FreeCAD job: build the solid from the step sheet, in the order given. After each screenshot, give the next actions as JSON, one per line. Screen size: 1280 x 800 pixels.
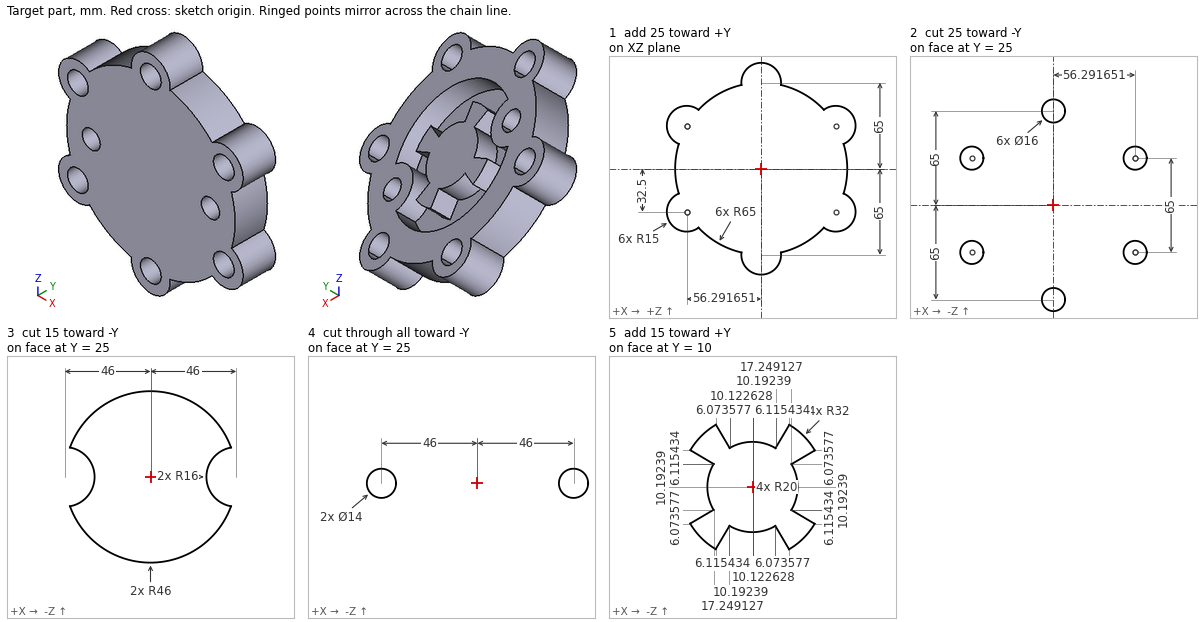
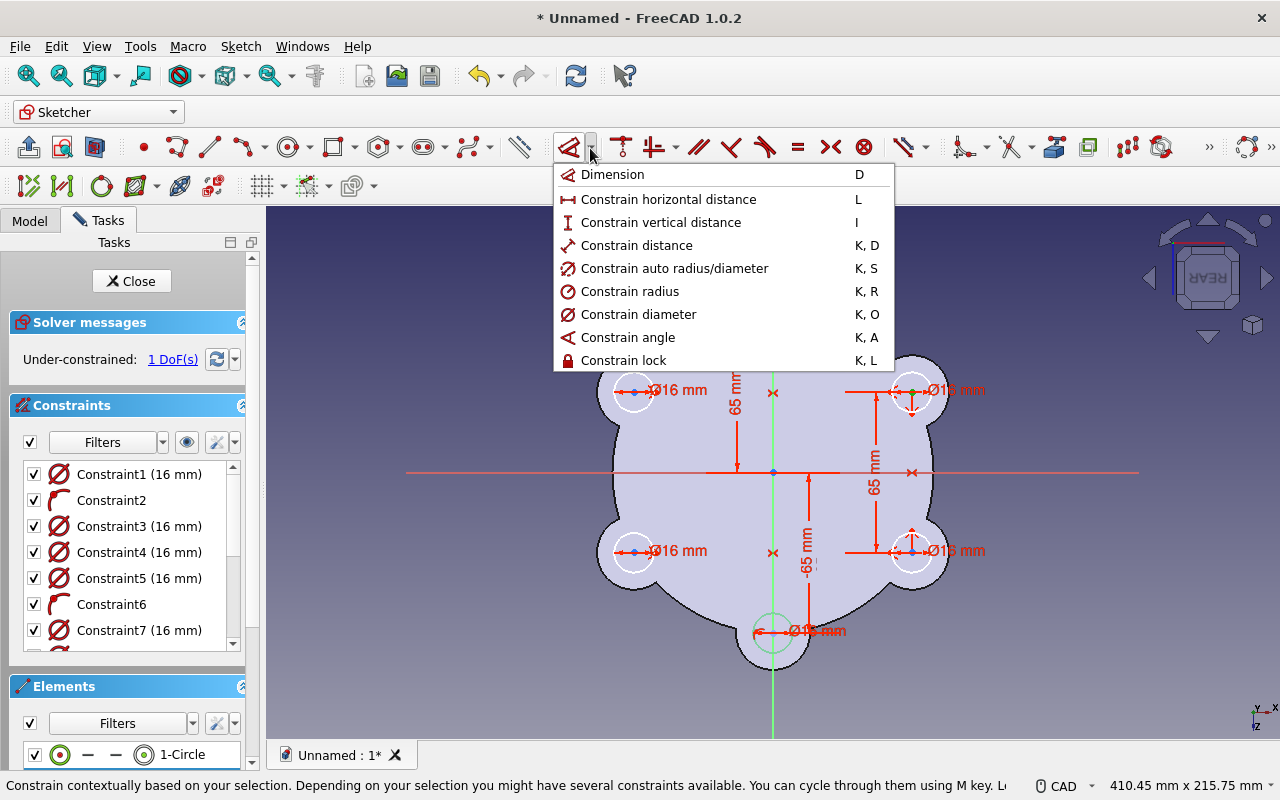
{"action": "left_click", "coordinate": [724, 200]}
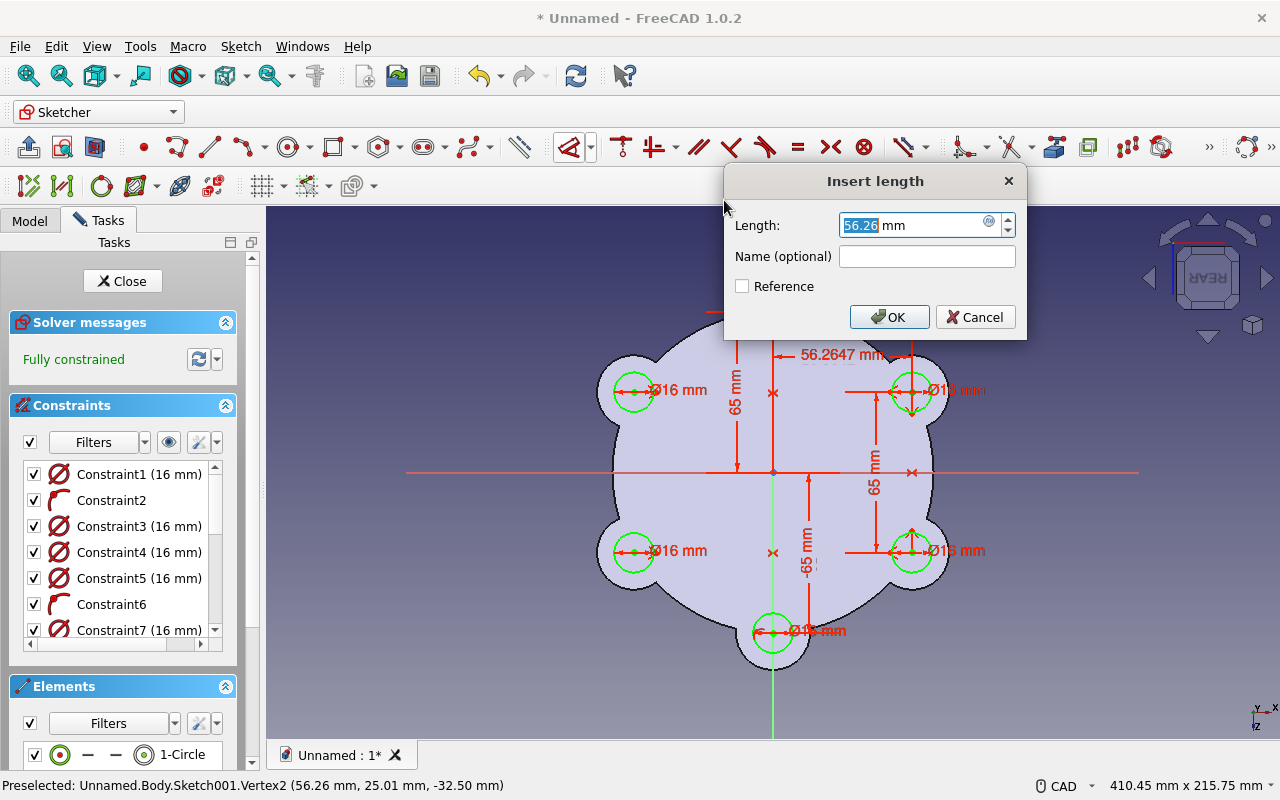
{"action": "type", "text": "56.291651"}
{"action": "key", "text": "Return"}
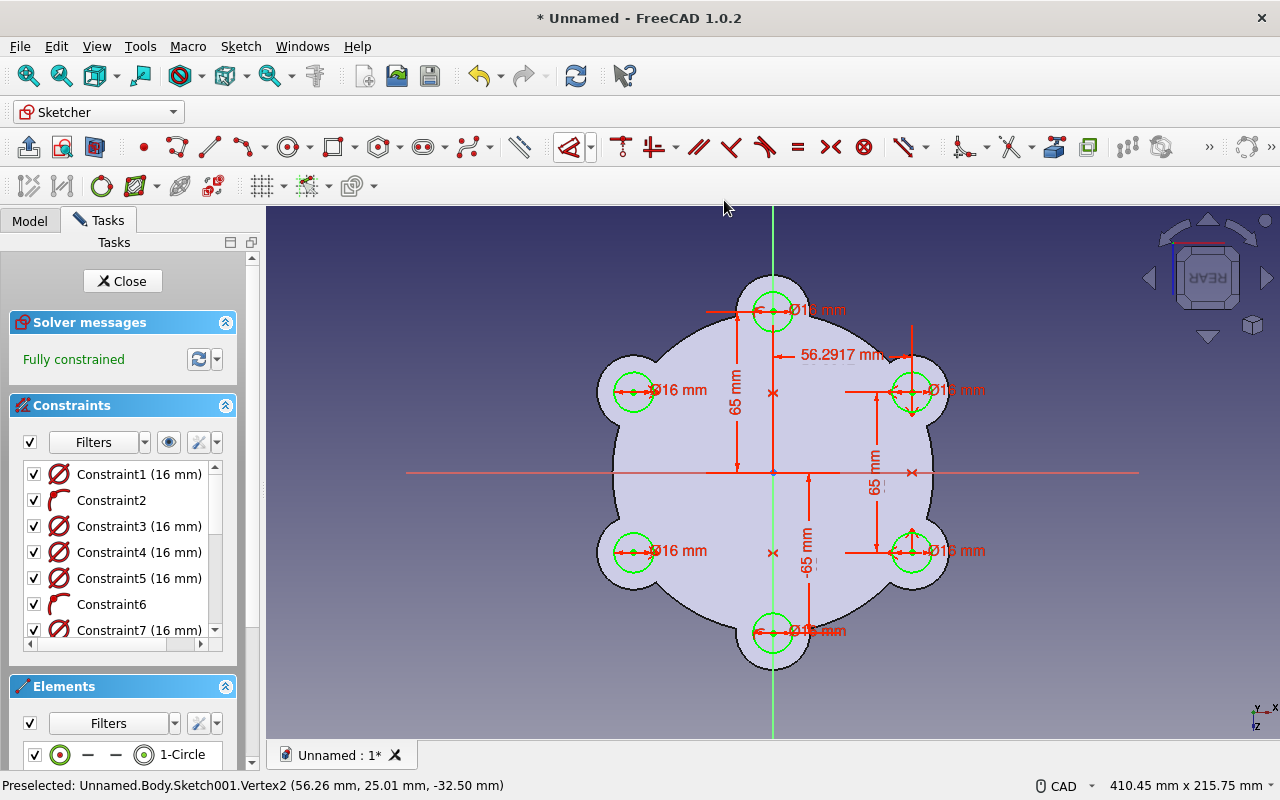
{"action": "left_click", "coordinate": [123, 281]}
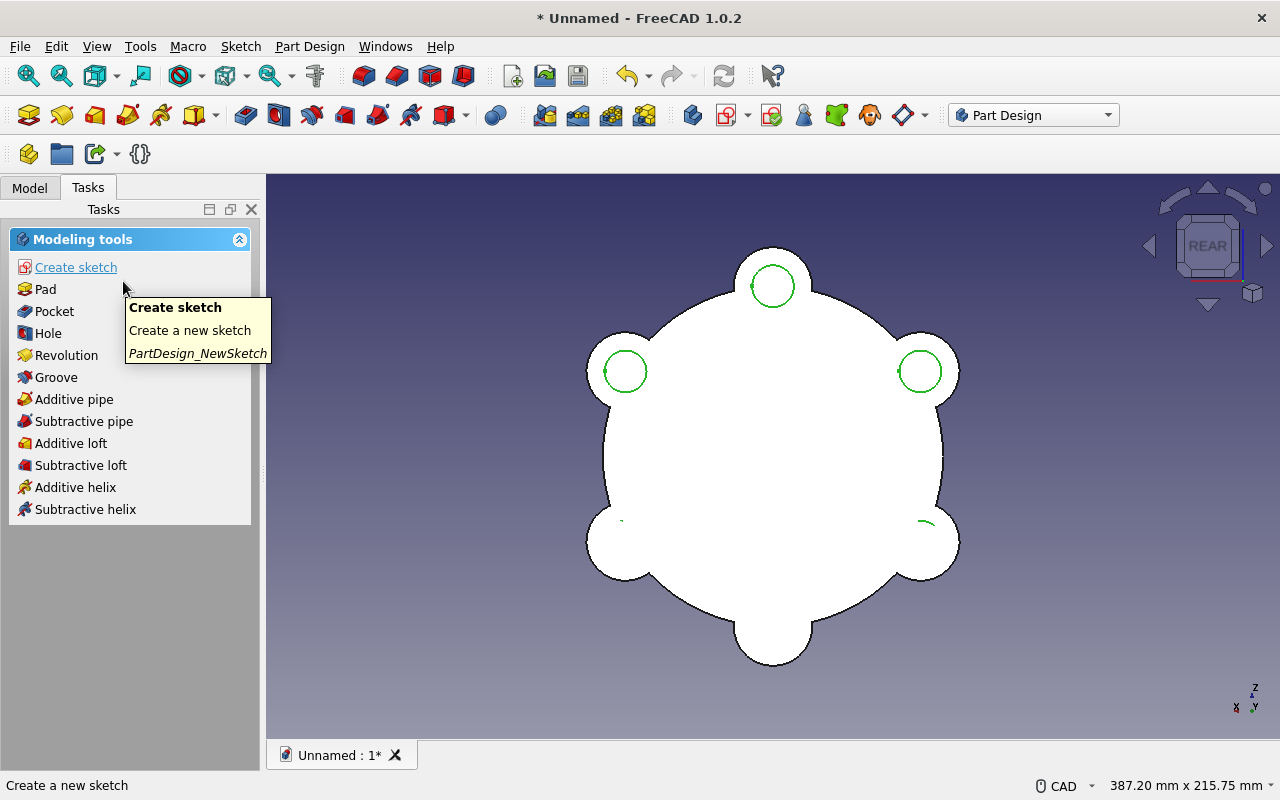
{"action": "left_click", "coordinate": [246, 116]}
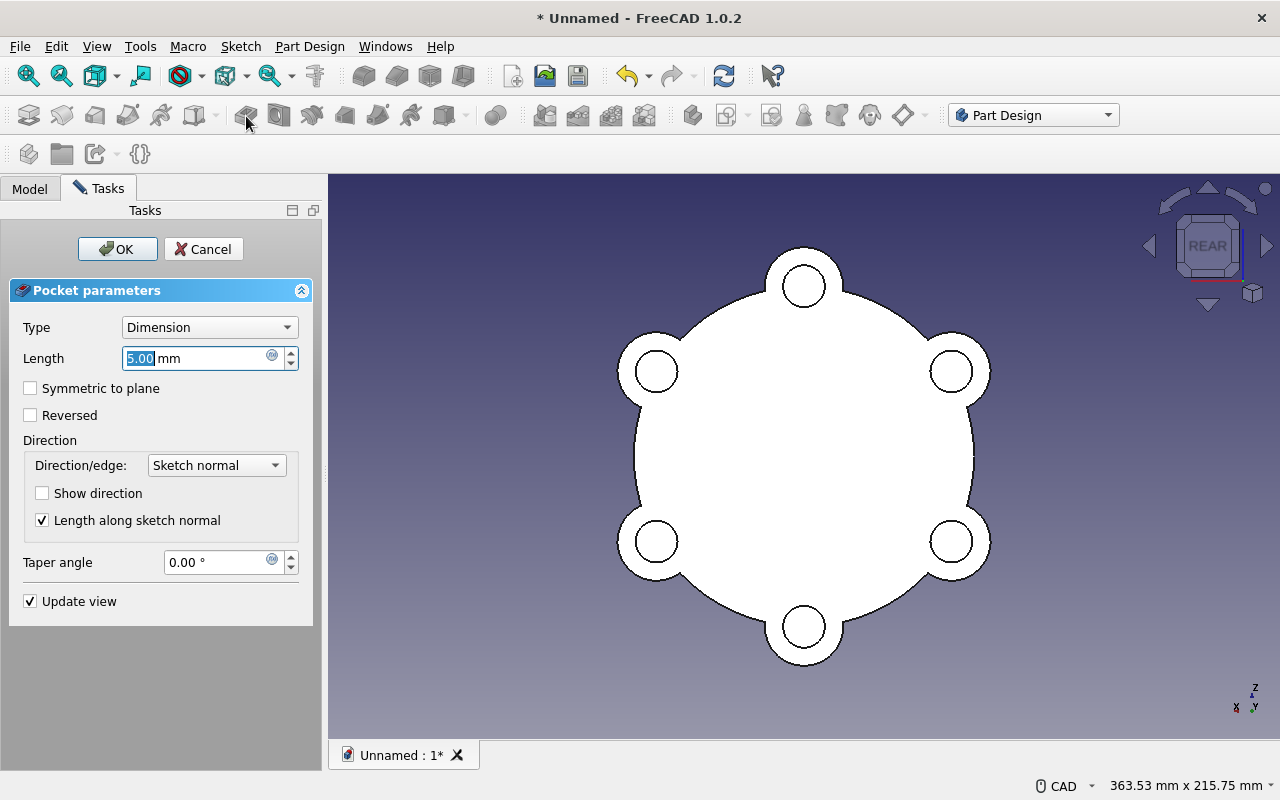
{"action": "type", "text": "25"}
{"action": "key", "text": "Tab"}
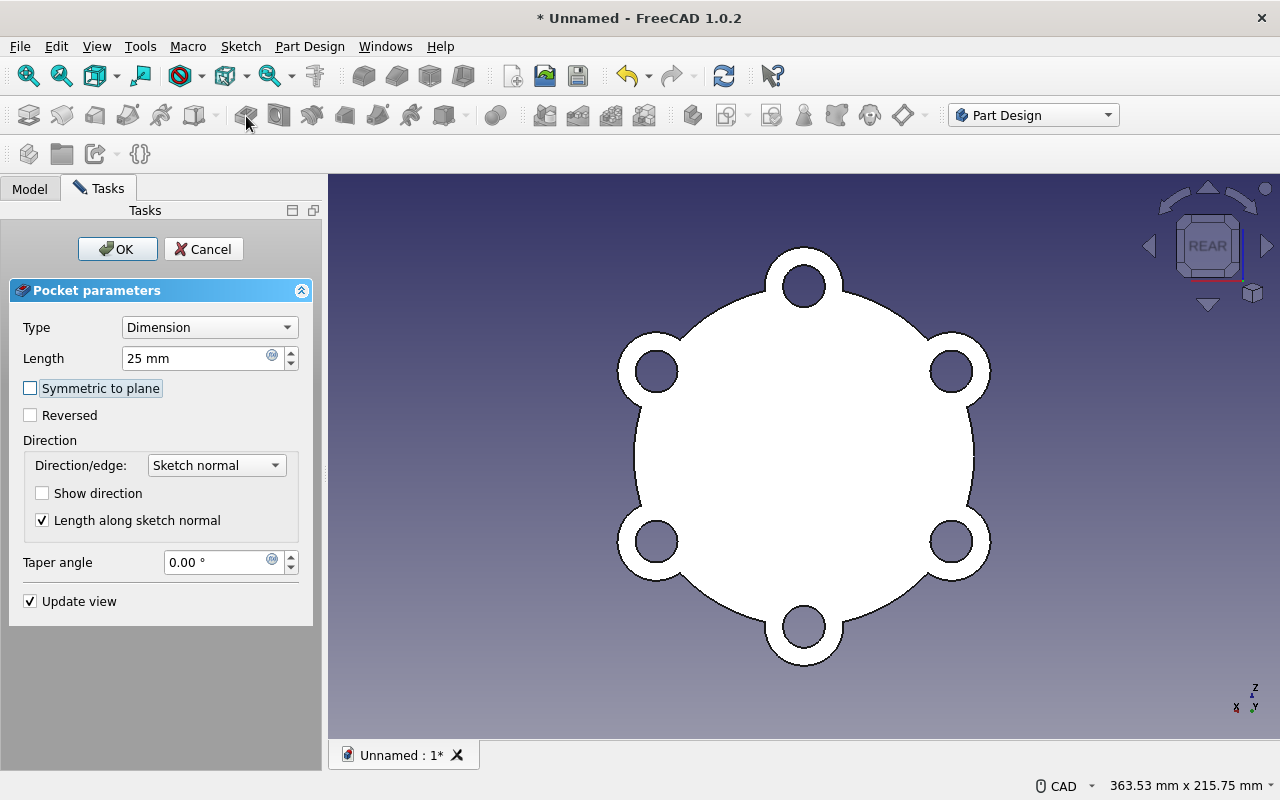
{"action": "left_click", "coordinate": [118, 249]}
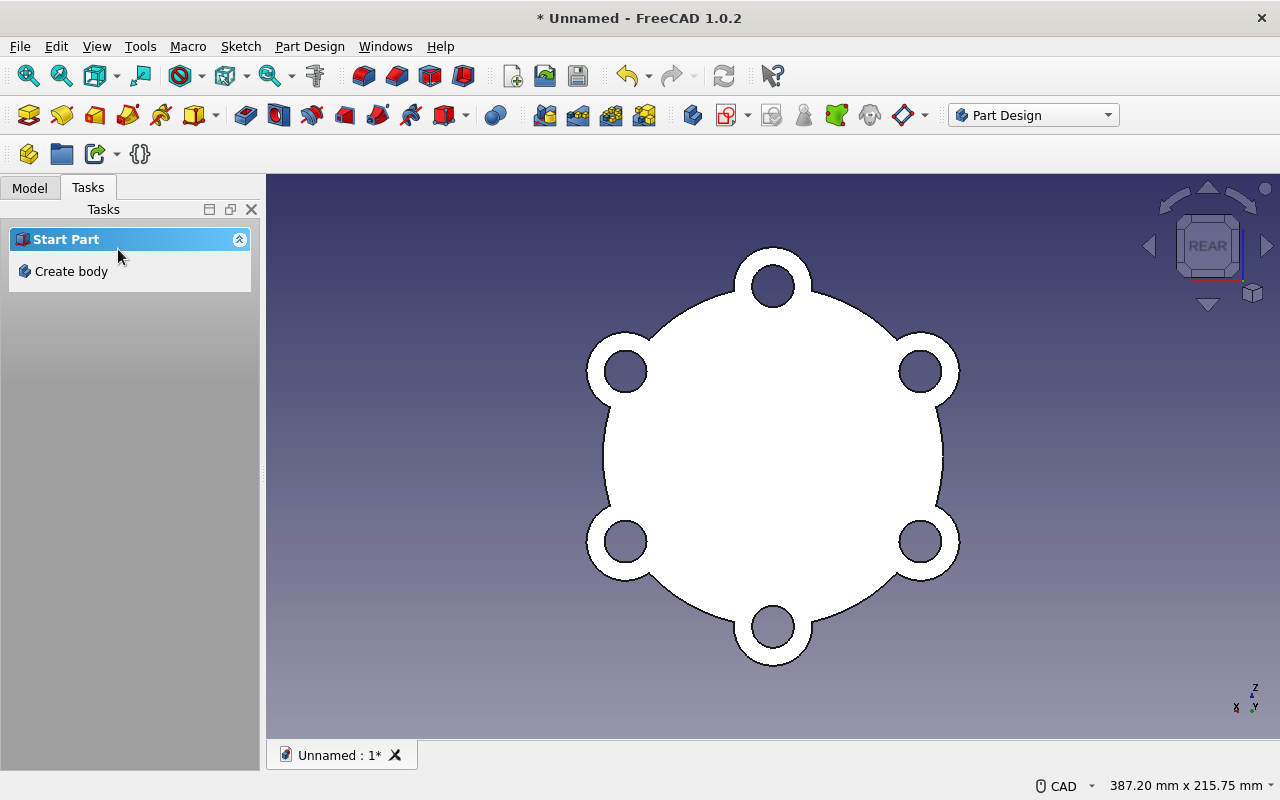
{"action": "left_click", "coordinate": [773, 455]}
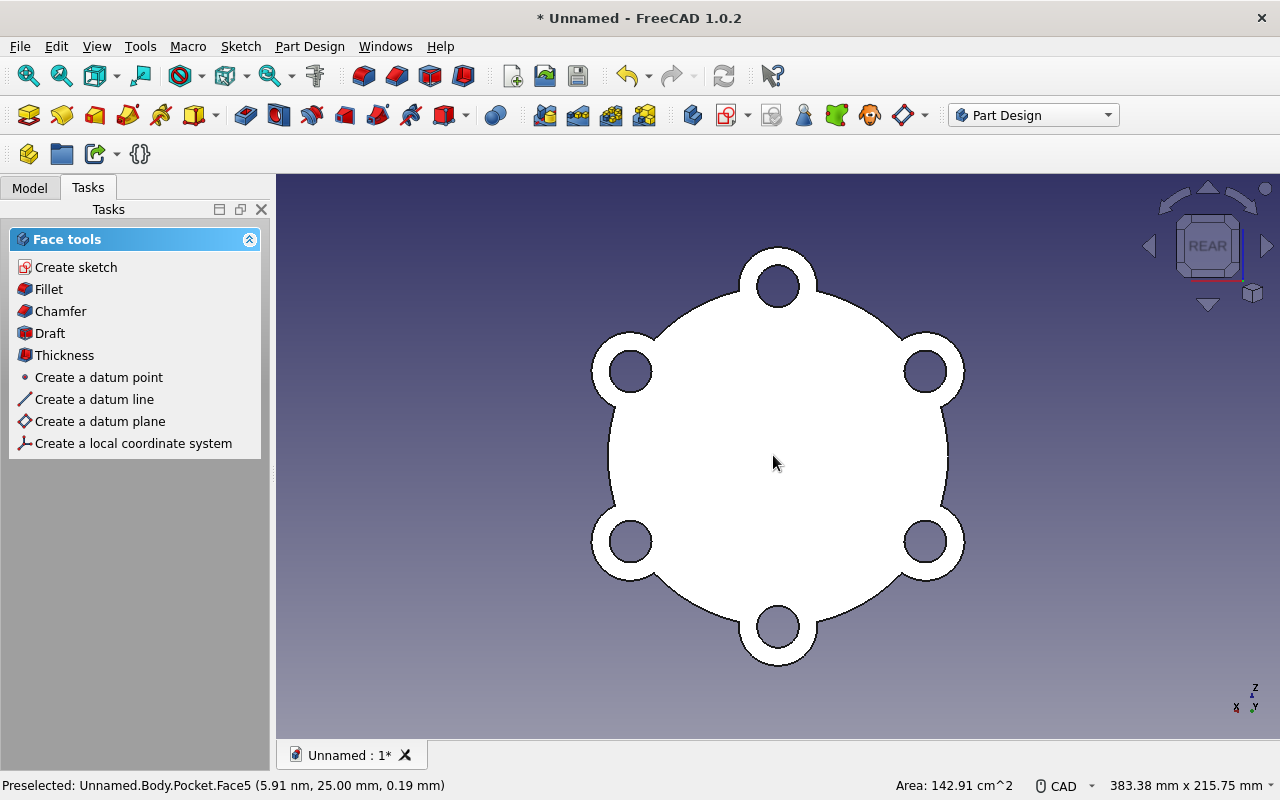
{"action": "left_click", "coordinate": [726, 116]}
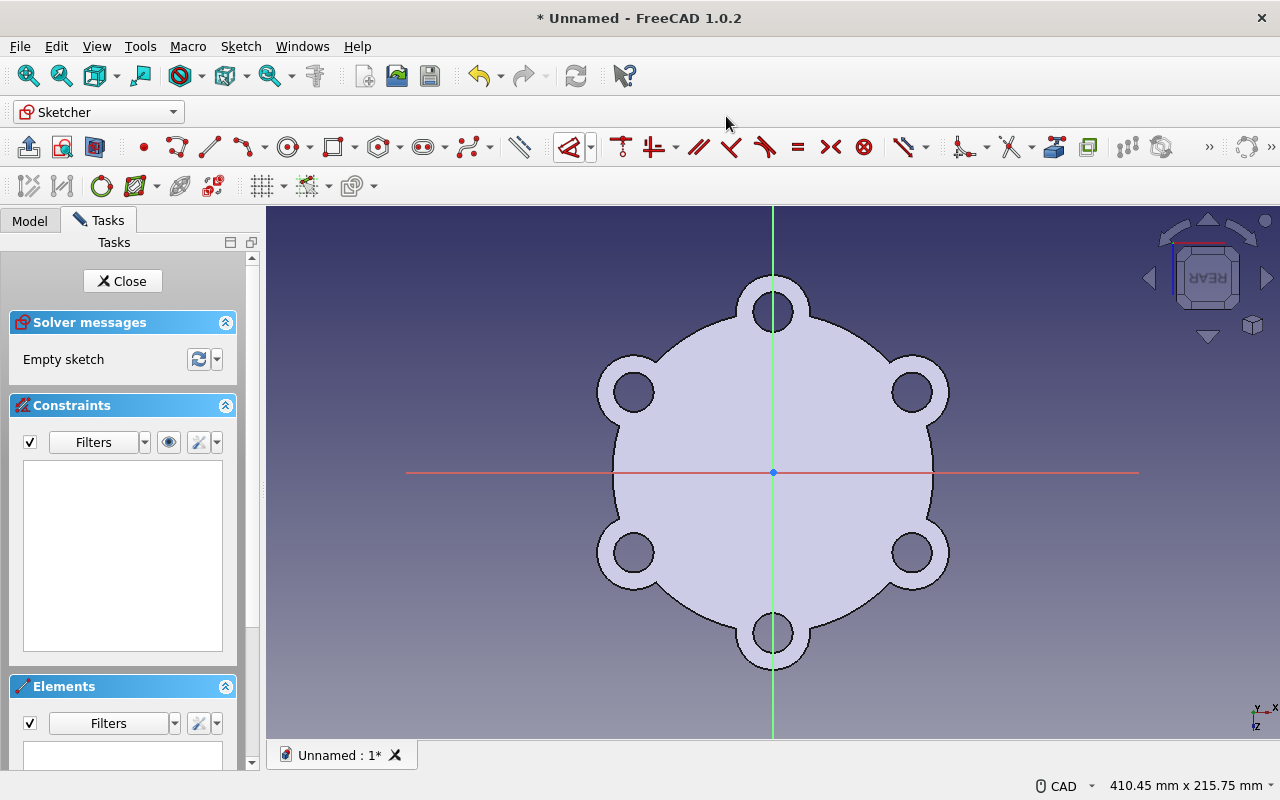
{"action": "scroll", "coordinate": [912, 472], "scroll_direction": "up", "scroll_amount": 2}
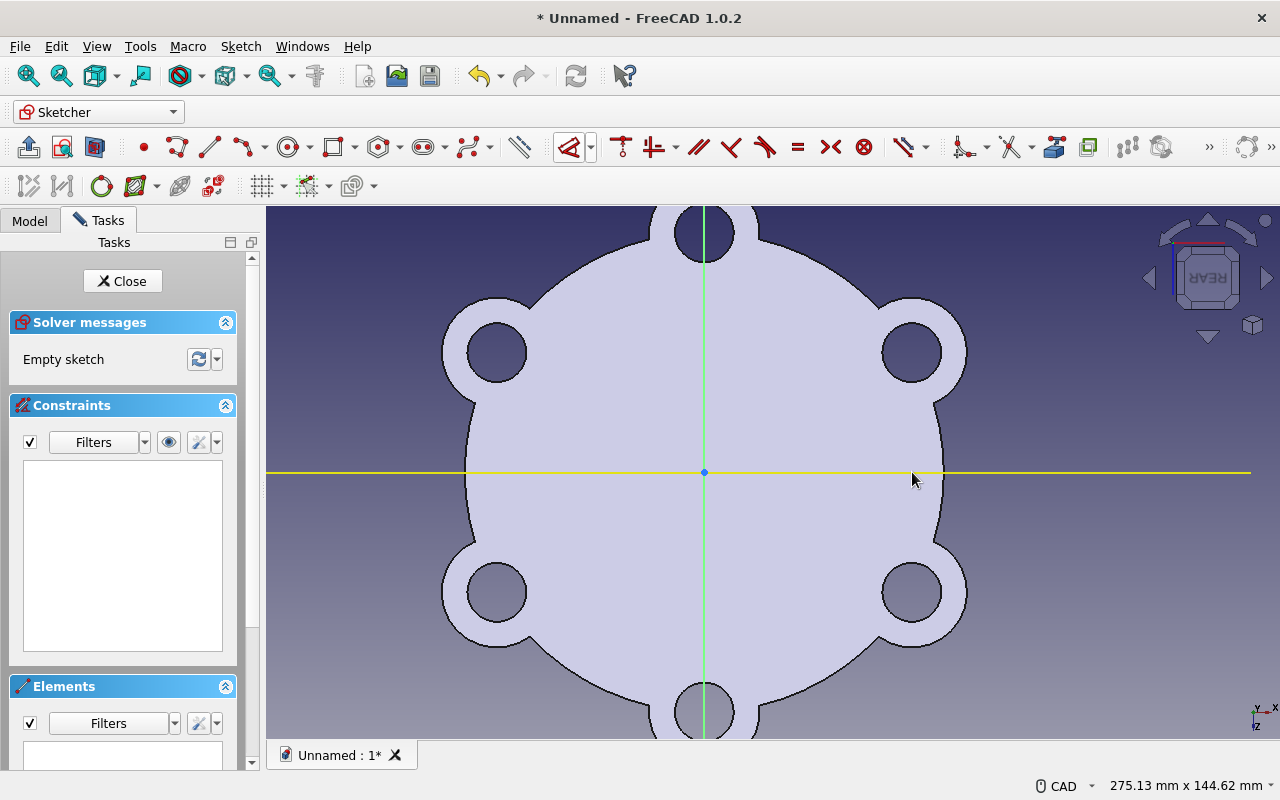
{"action": "left_click", "coordinate": [242, 148]}